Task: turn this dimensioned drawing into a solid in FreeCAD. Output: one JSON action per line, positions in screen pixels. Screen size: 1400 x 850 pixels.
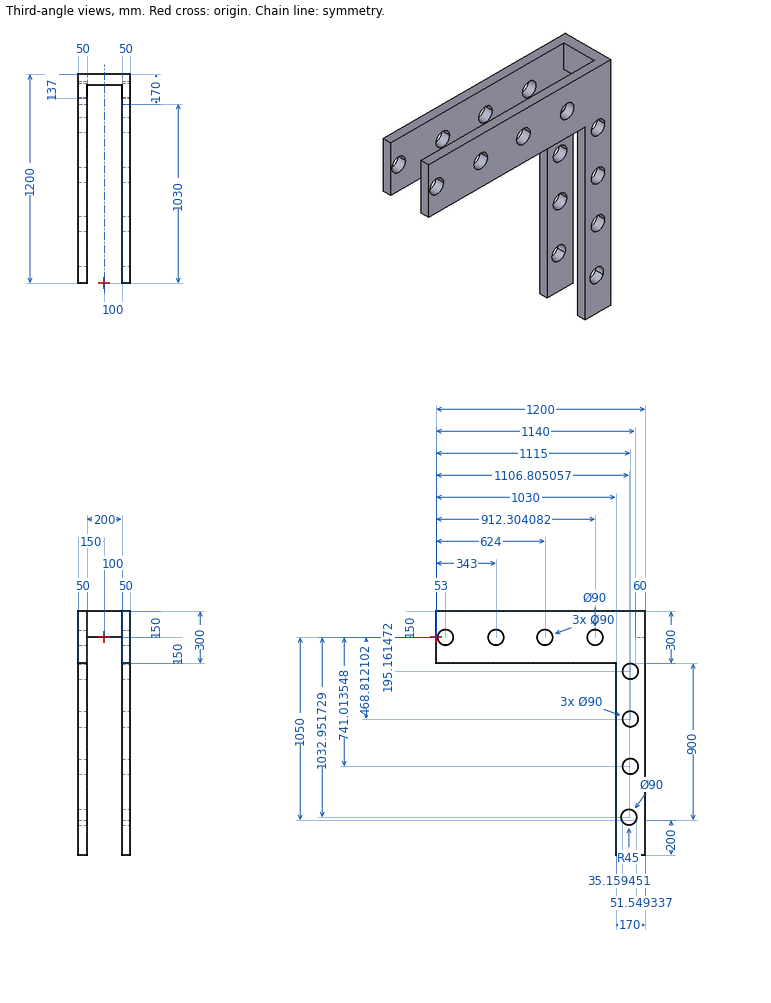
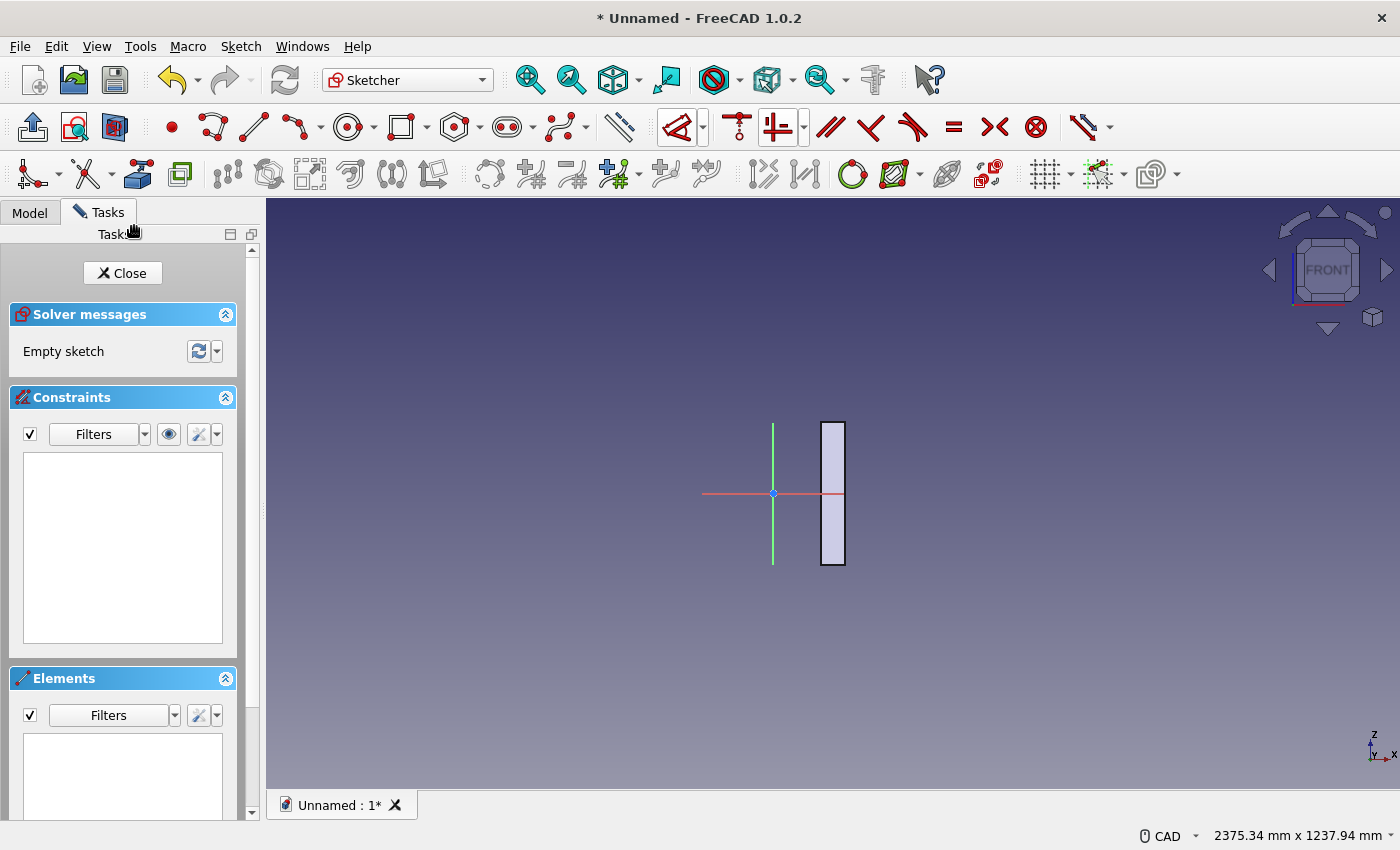
{"action": "scroll", "coordinate": [722, 494], "scroll_direction": "up", "scroll_amount": 5}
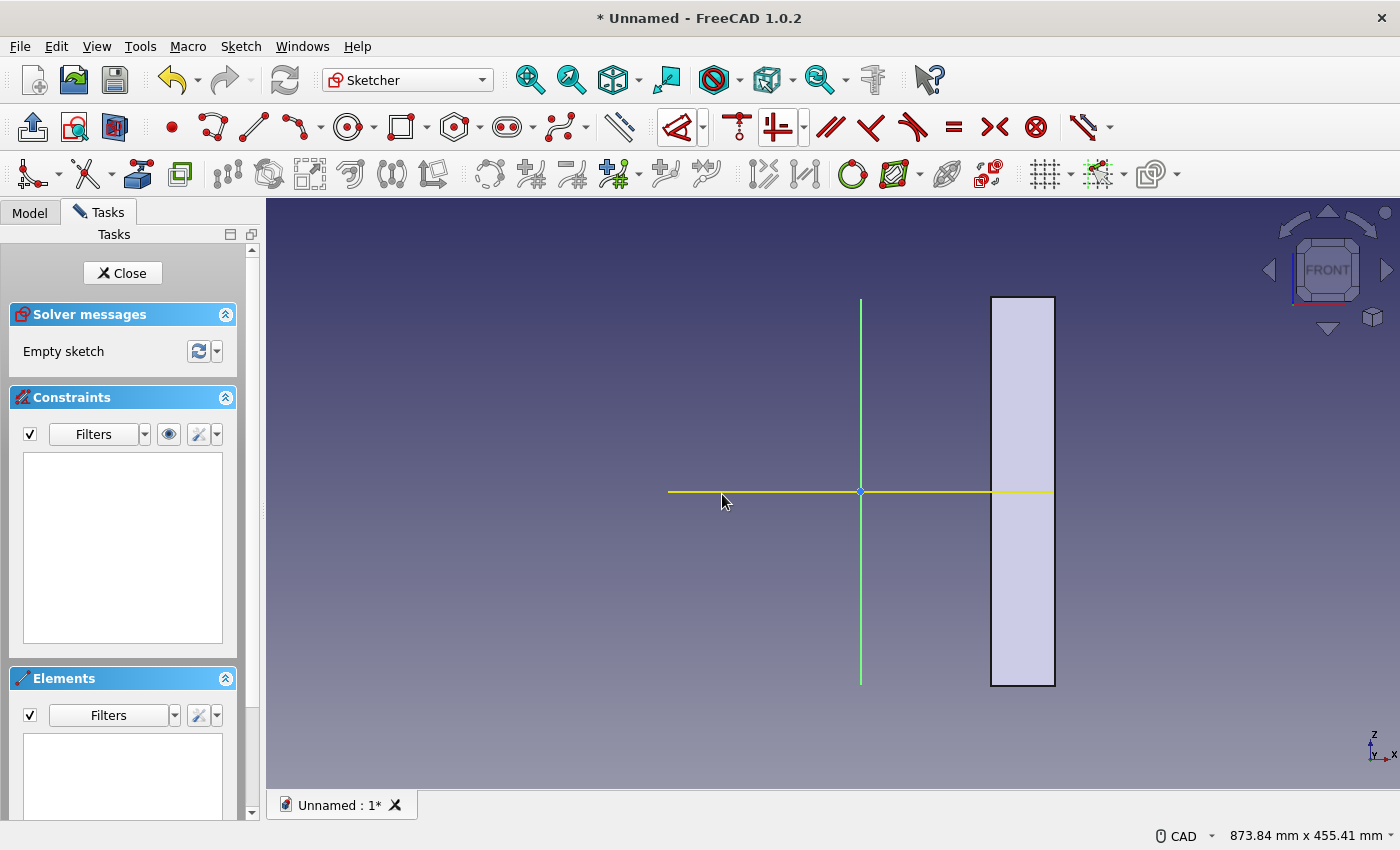
{"action": "left_click", "coordinate": [400, 128]}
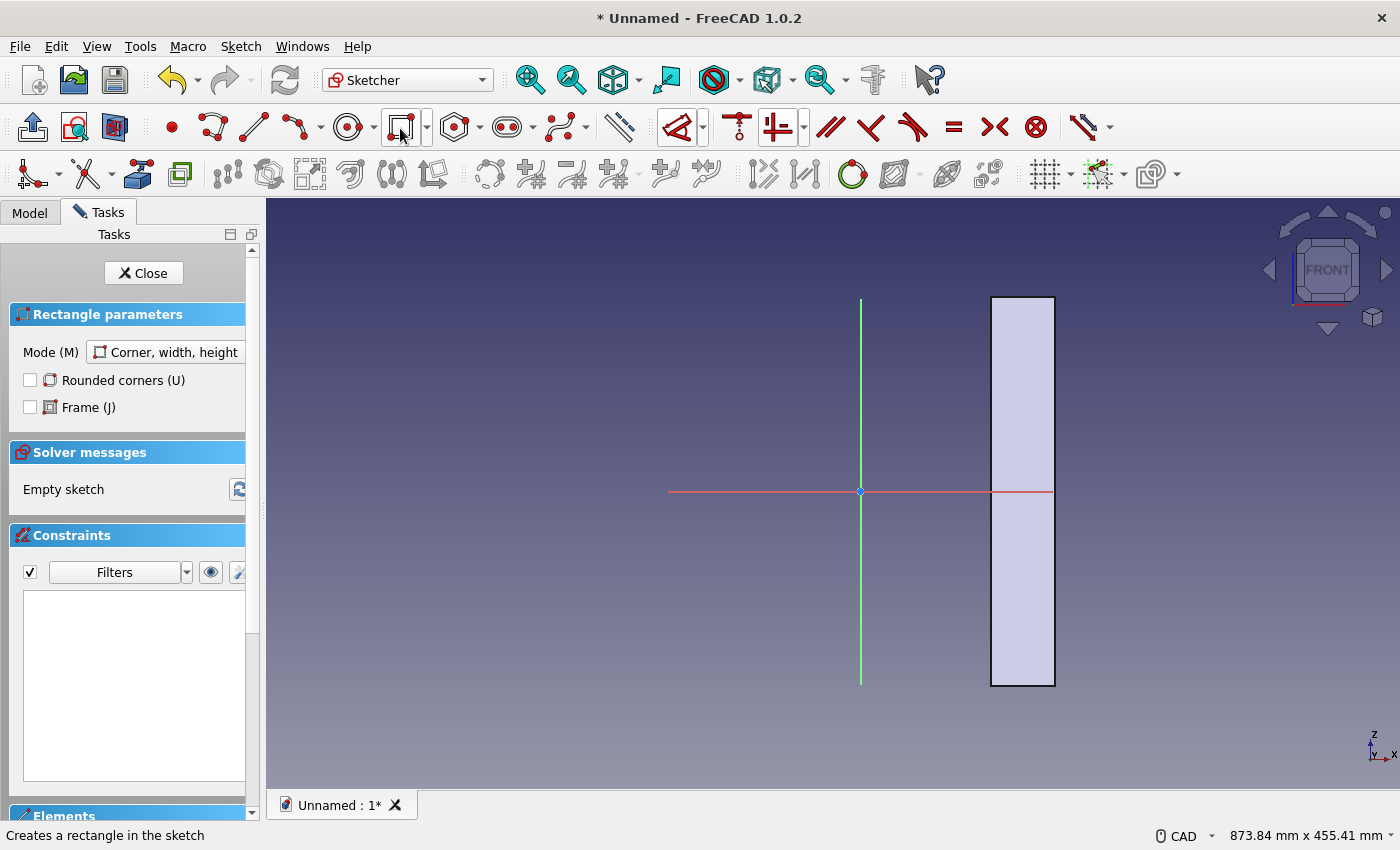
{"action": "left_click", "coordinate": [666, 297]}
{"action": "left_click", "coordinate": [731, 686]}
{"action": "key", "text": "Escape"}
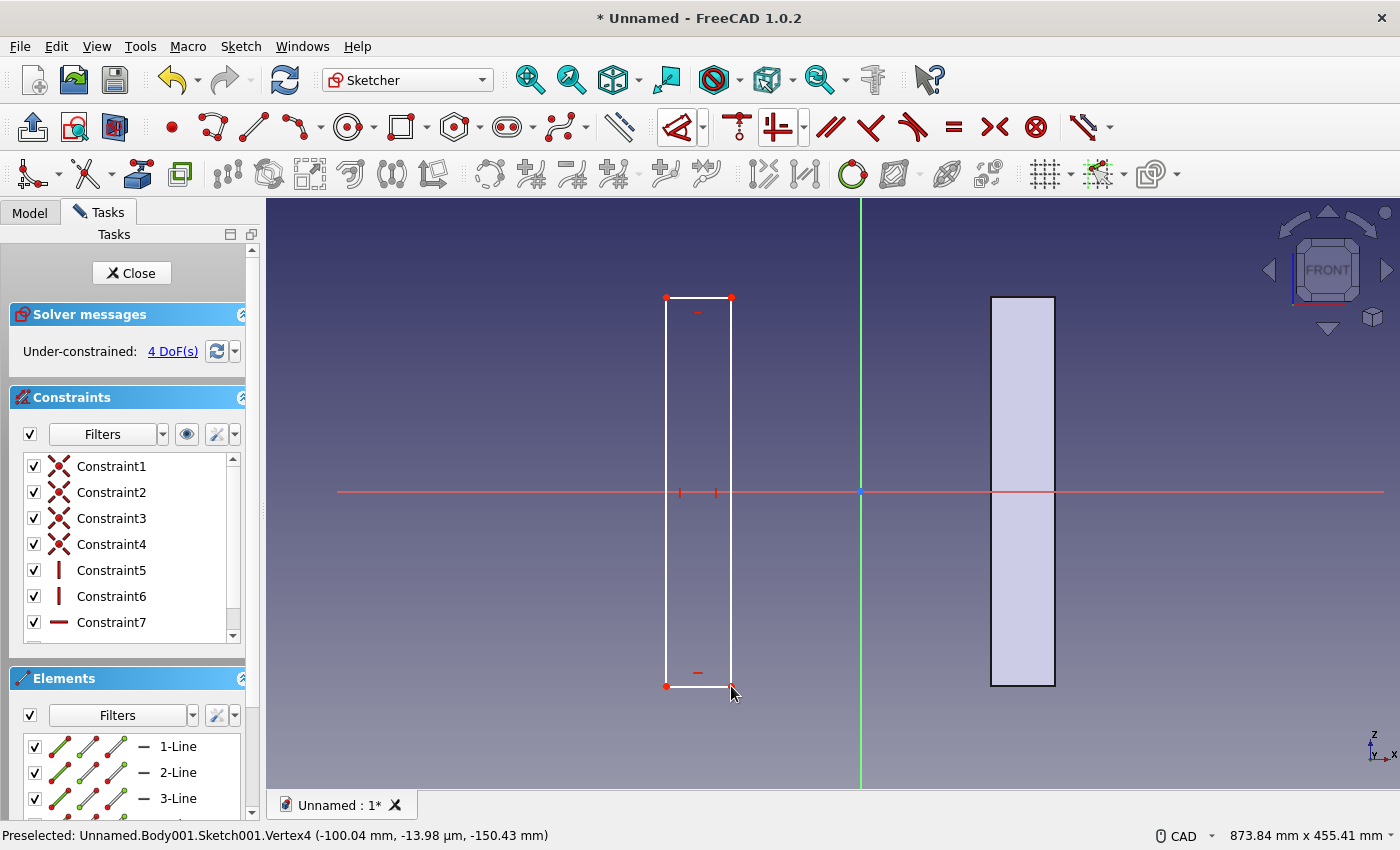
{"action": "left_click", "coordinate": [685, 687]}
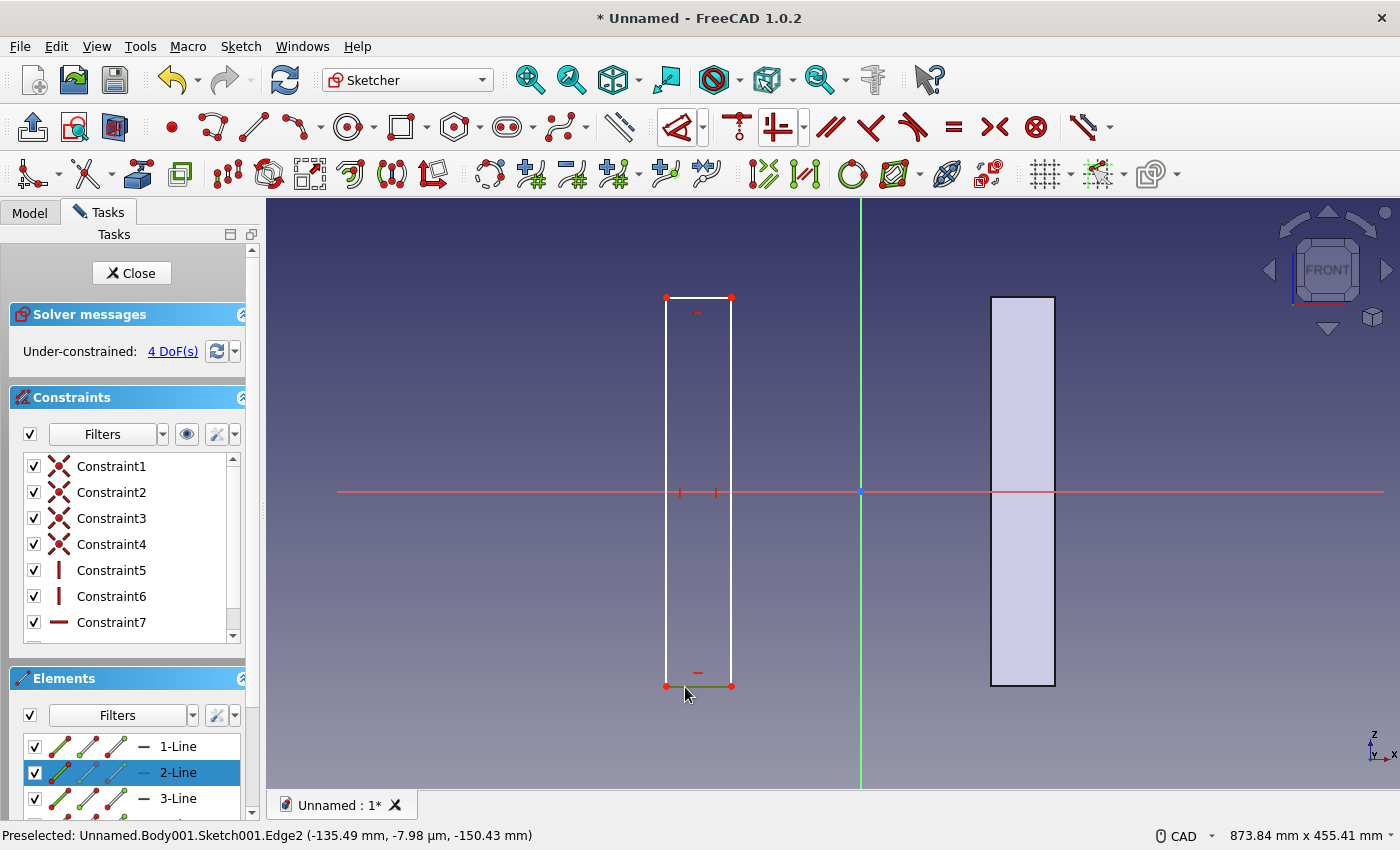
{"action": "left_click", "coordinate": [702, 128]}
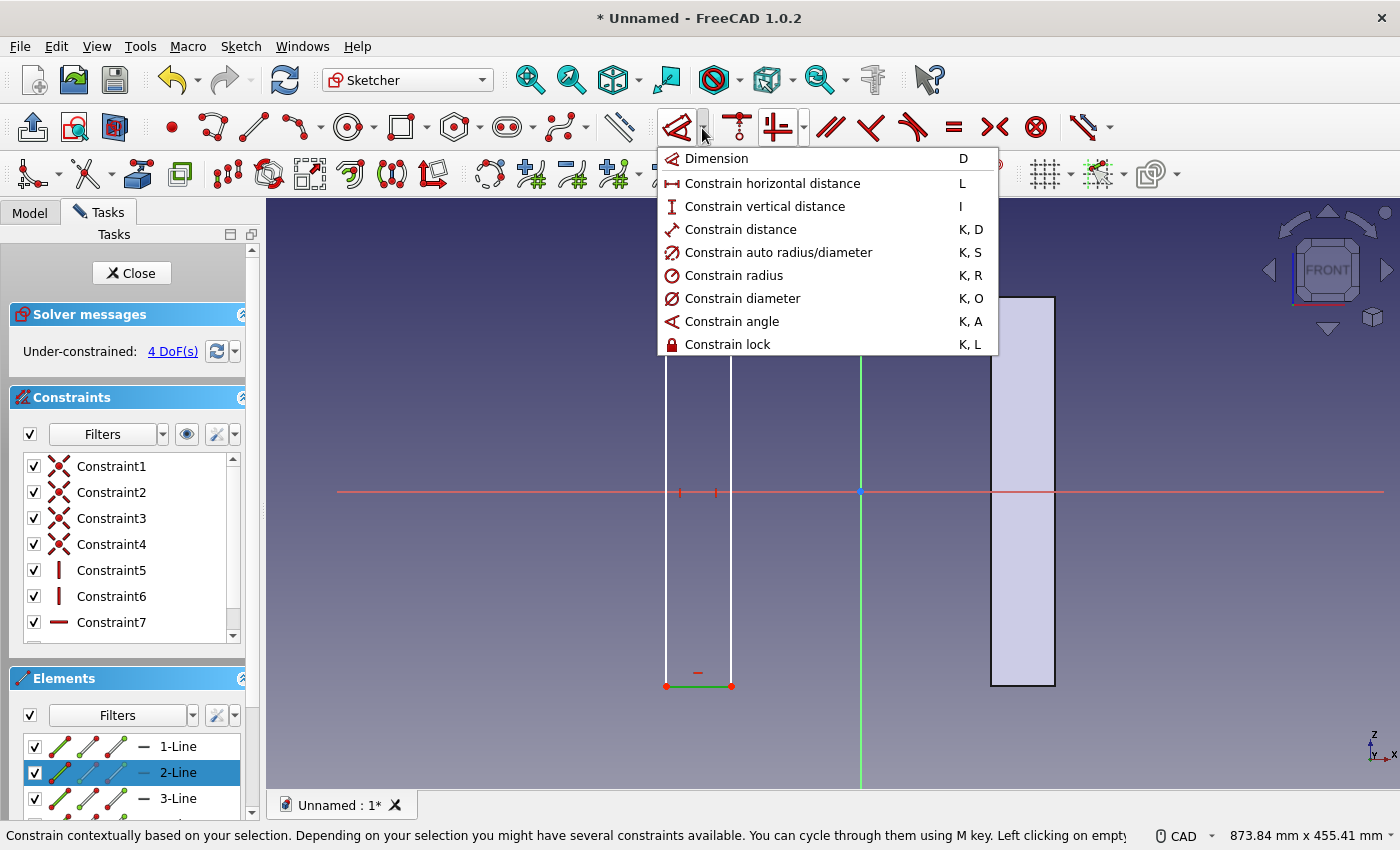
{"action": "left_click", "coordinate": [828, 184]}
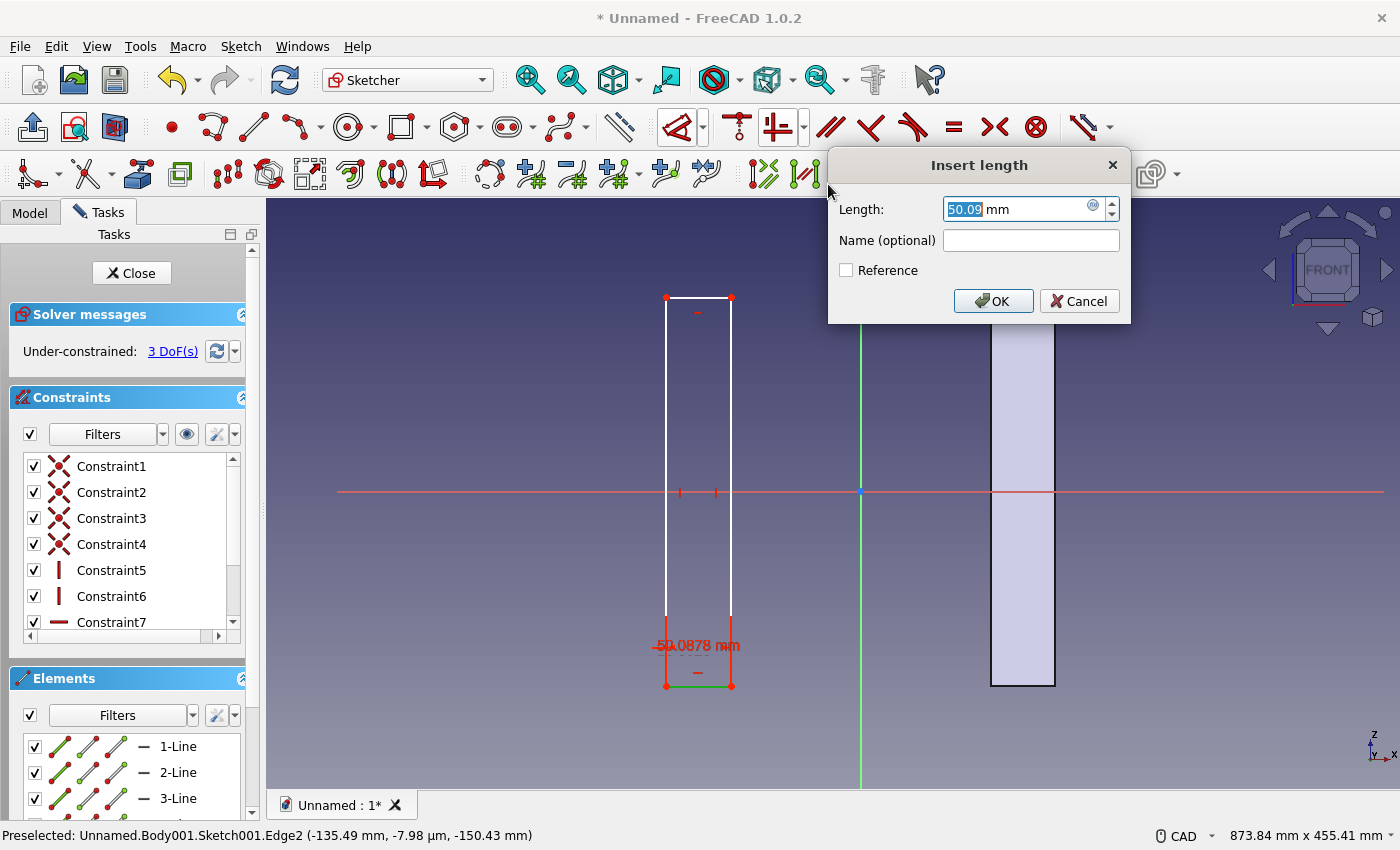
{"action": "type", "text": "50"}
{"action": "key", "text": "Return"}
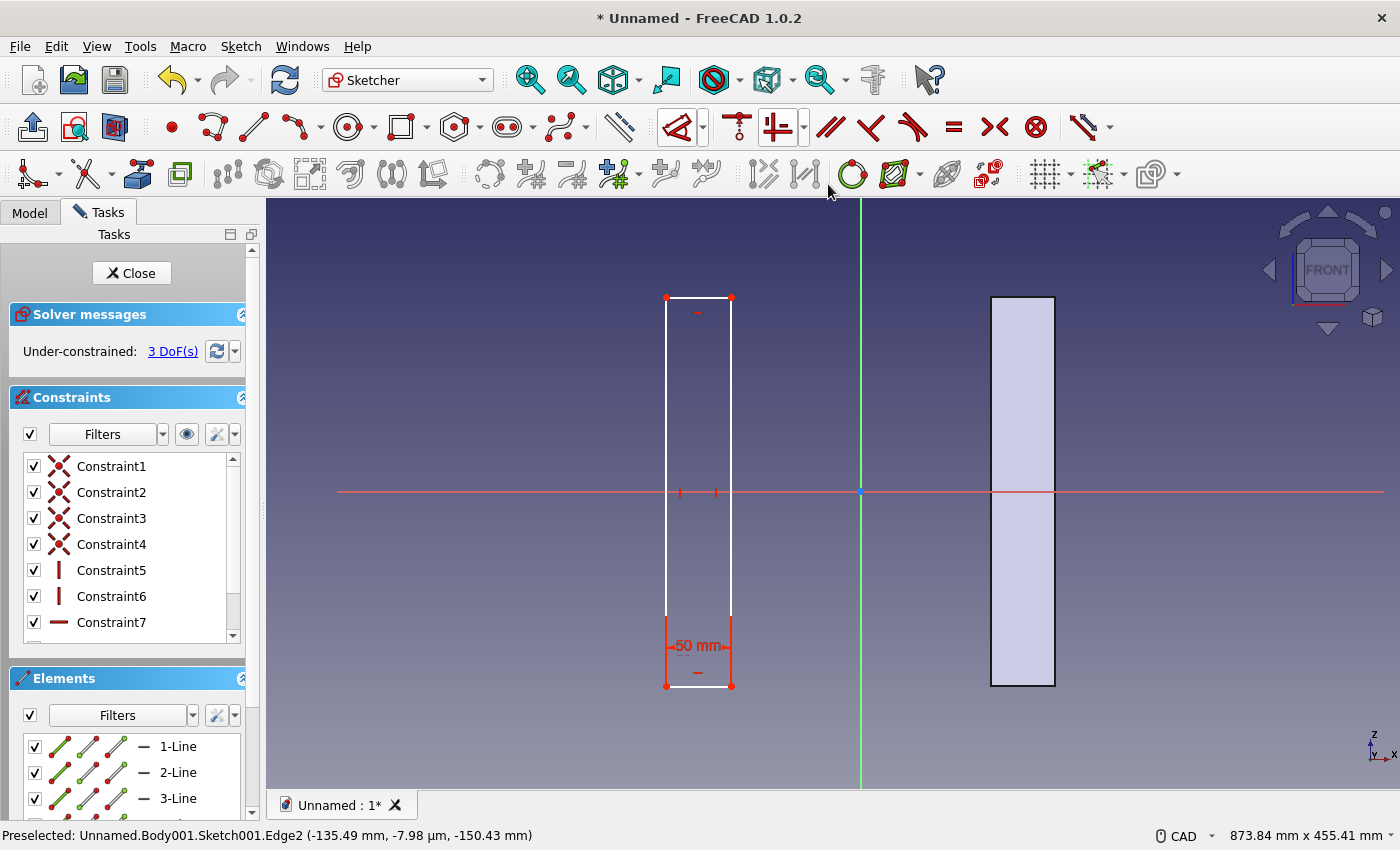
{"action": "left_click", "coordinate": [666, 415]}